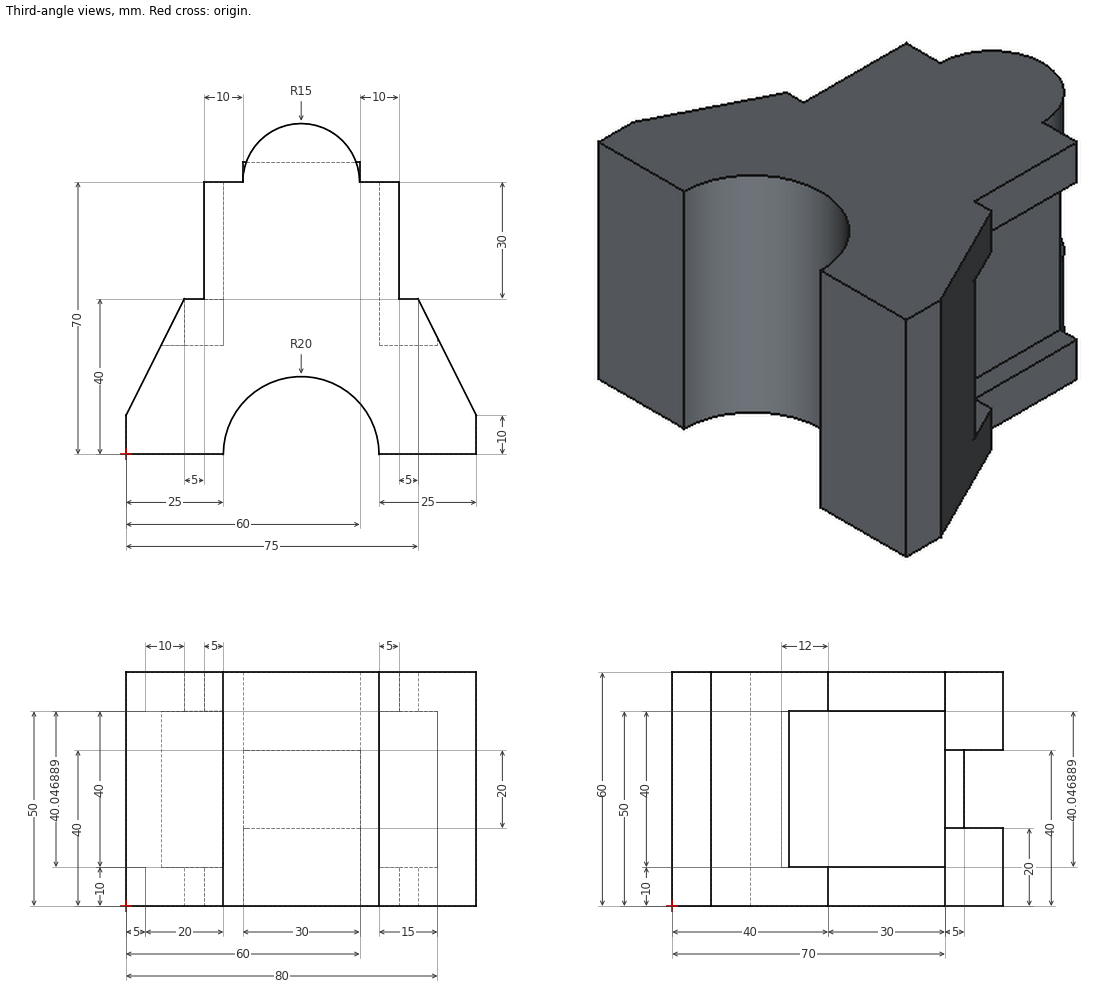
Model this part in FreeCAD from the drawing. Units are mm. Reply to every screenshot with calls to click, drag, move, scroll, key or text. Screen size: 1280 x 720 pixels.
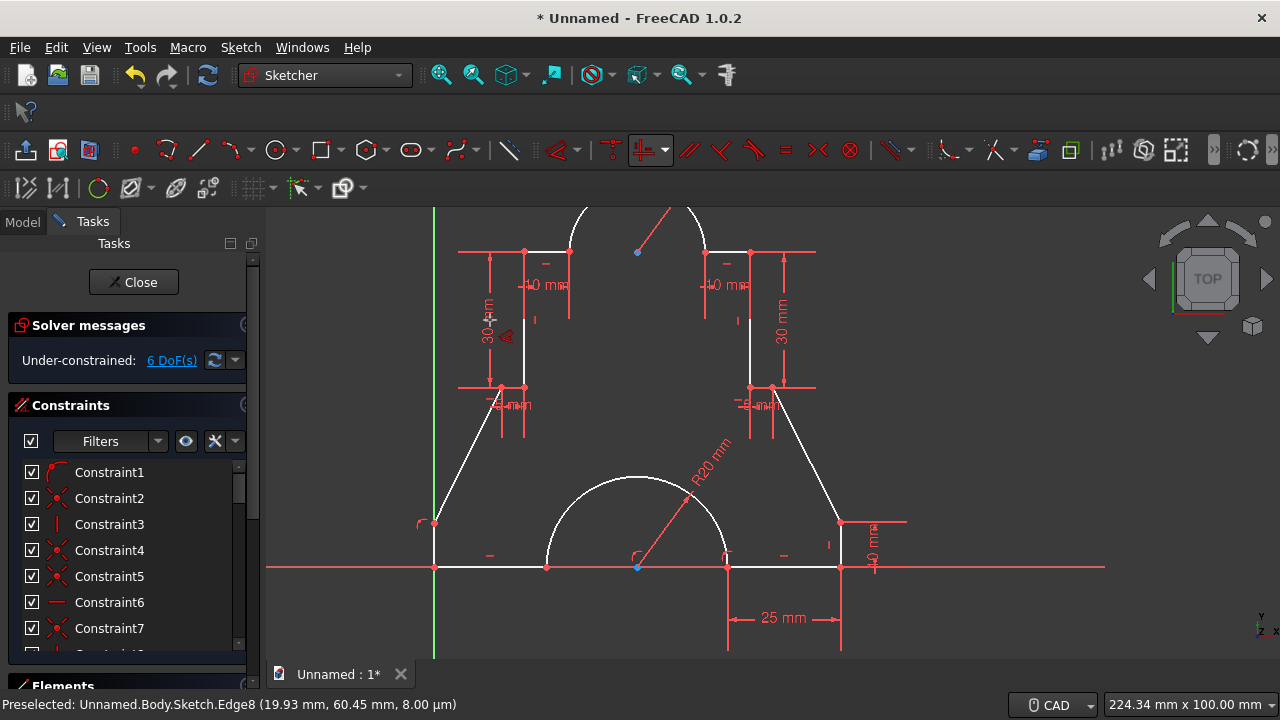
click(434, 536)
click(400, 545)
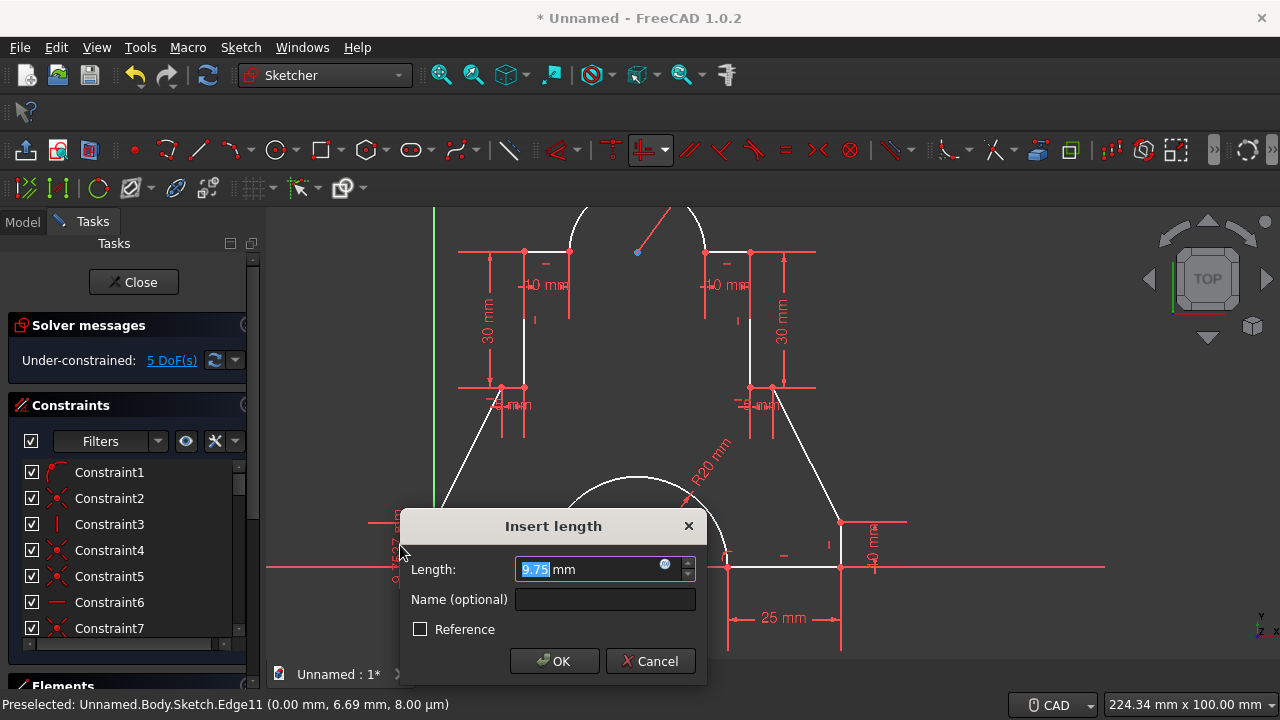
text(10)
key(Return)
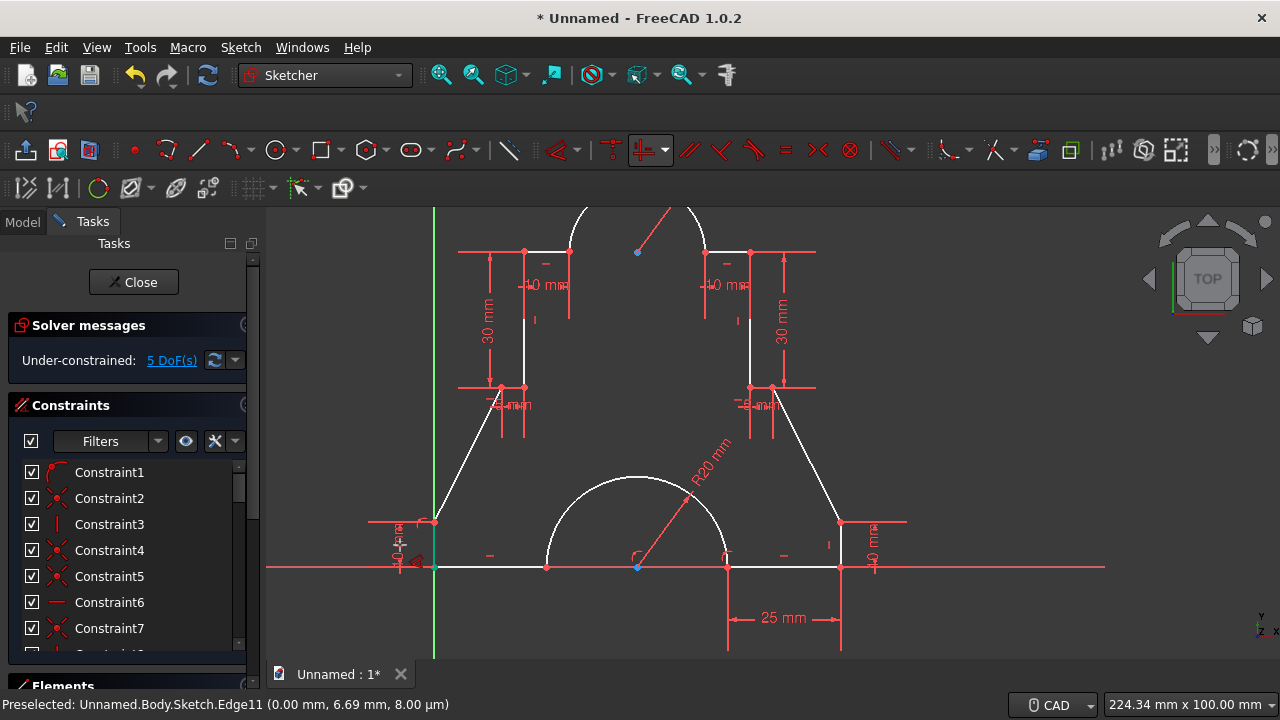
click(468, 567)
click(490, 601)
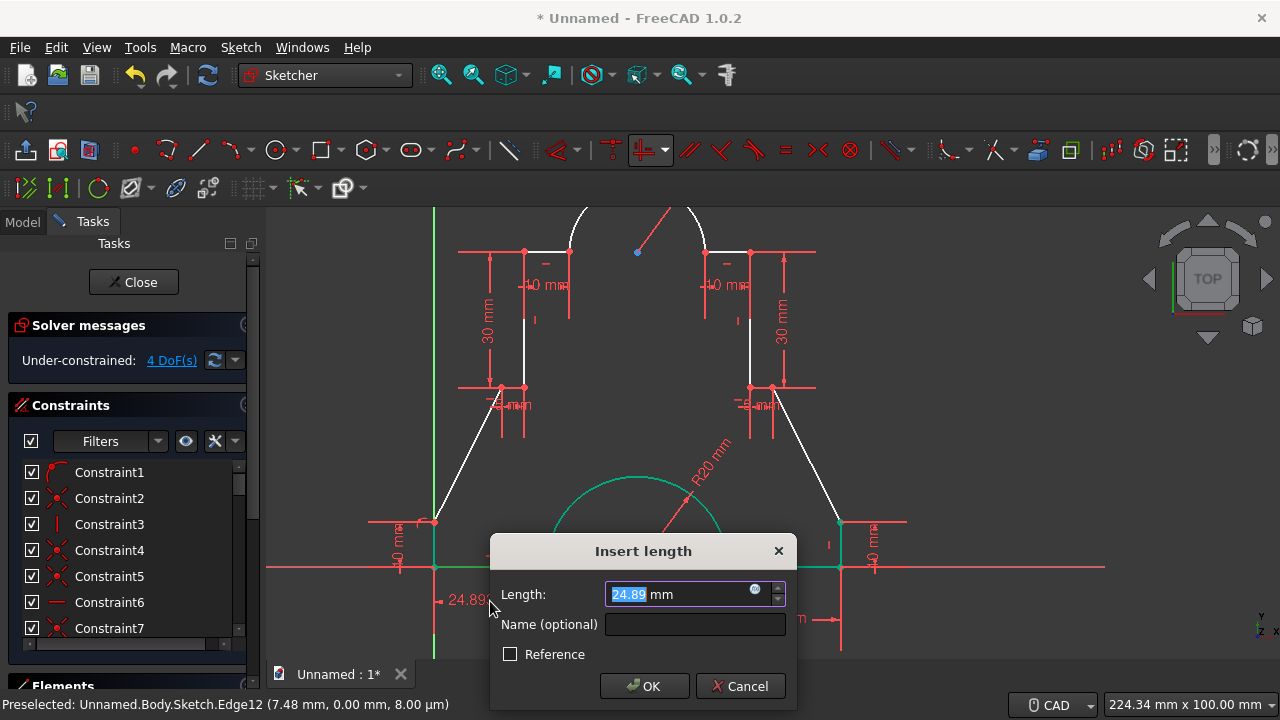
text(25)
key(Return)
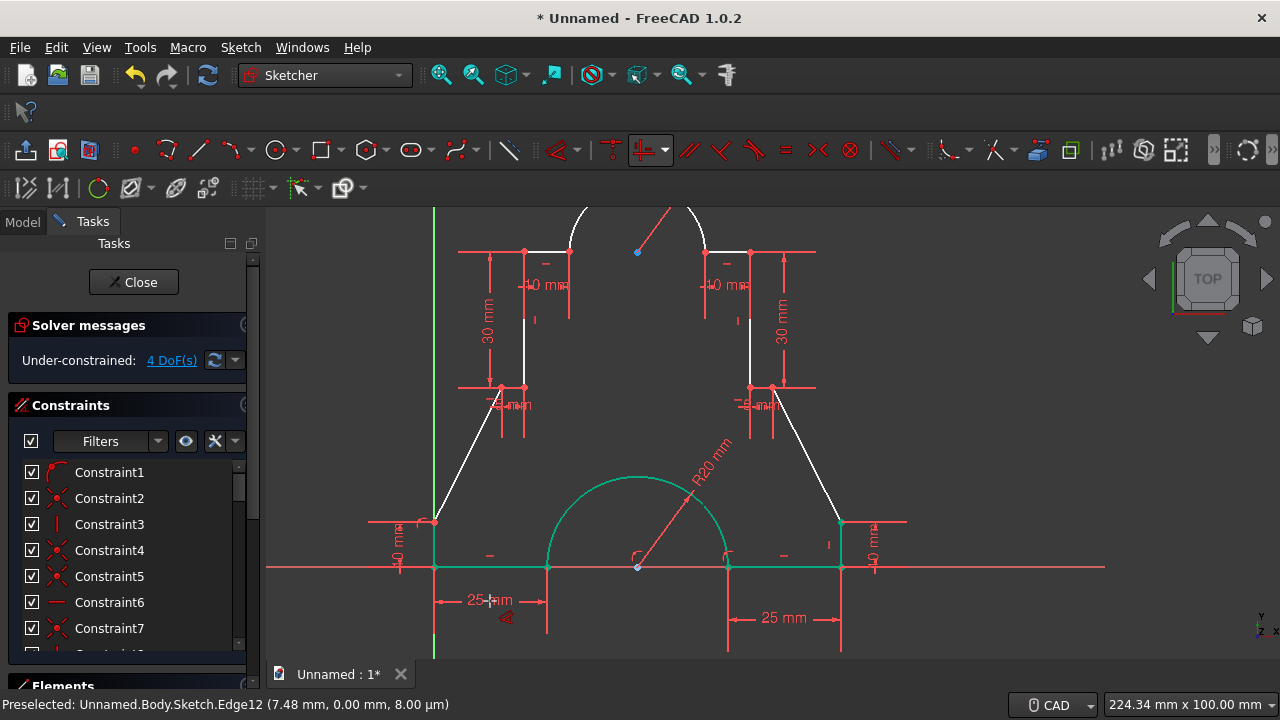
click(773, 388)
click(604, 601)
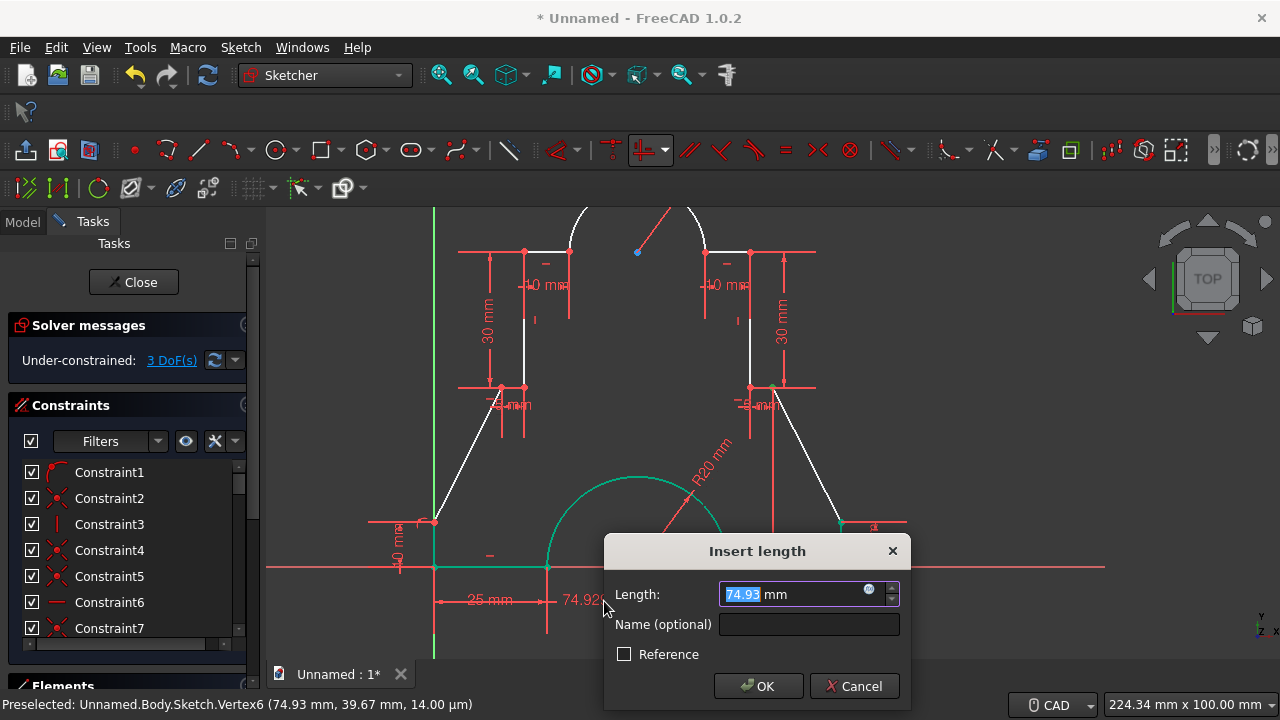
text(75)
key(Return)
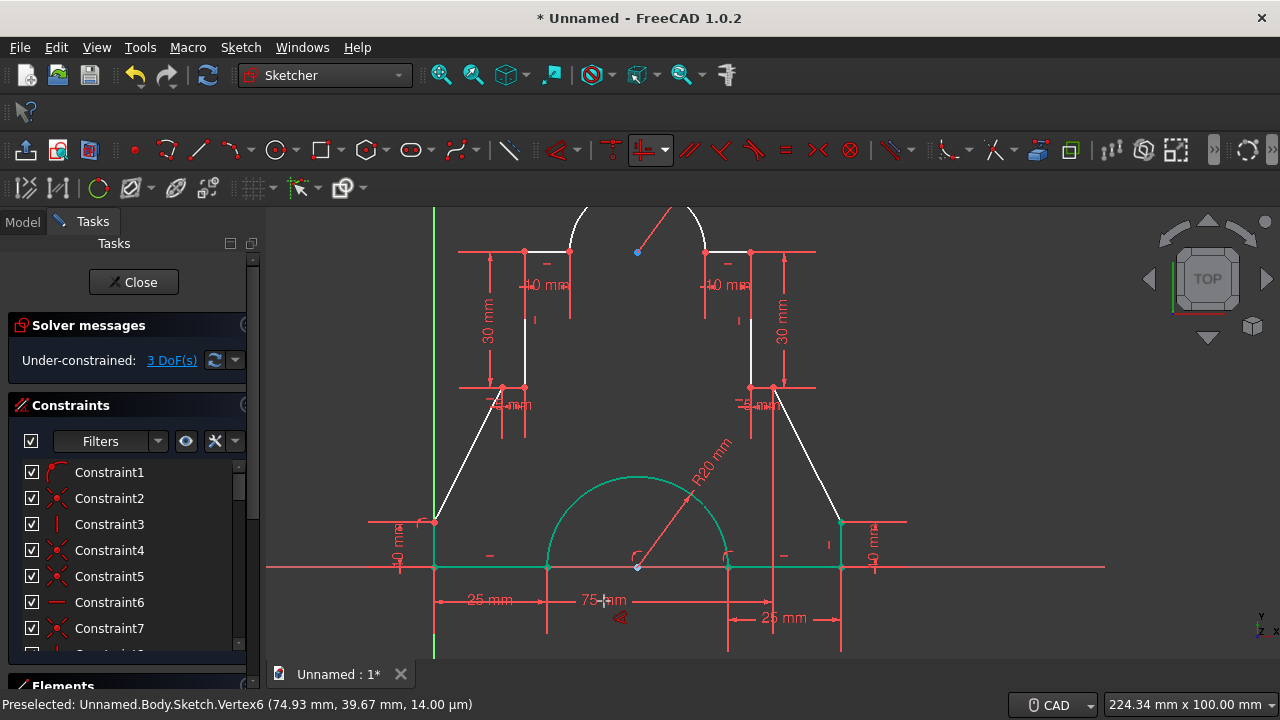
click(773, 388)
click(400, 478)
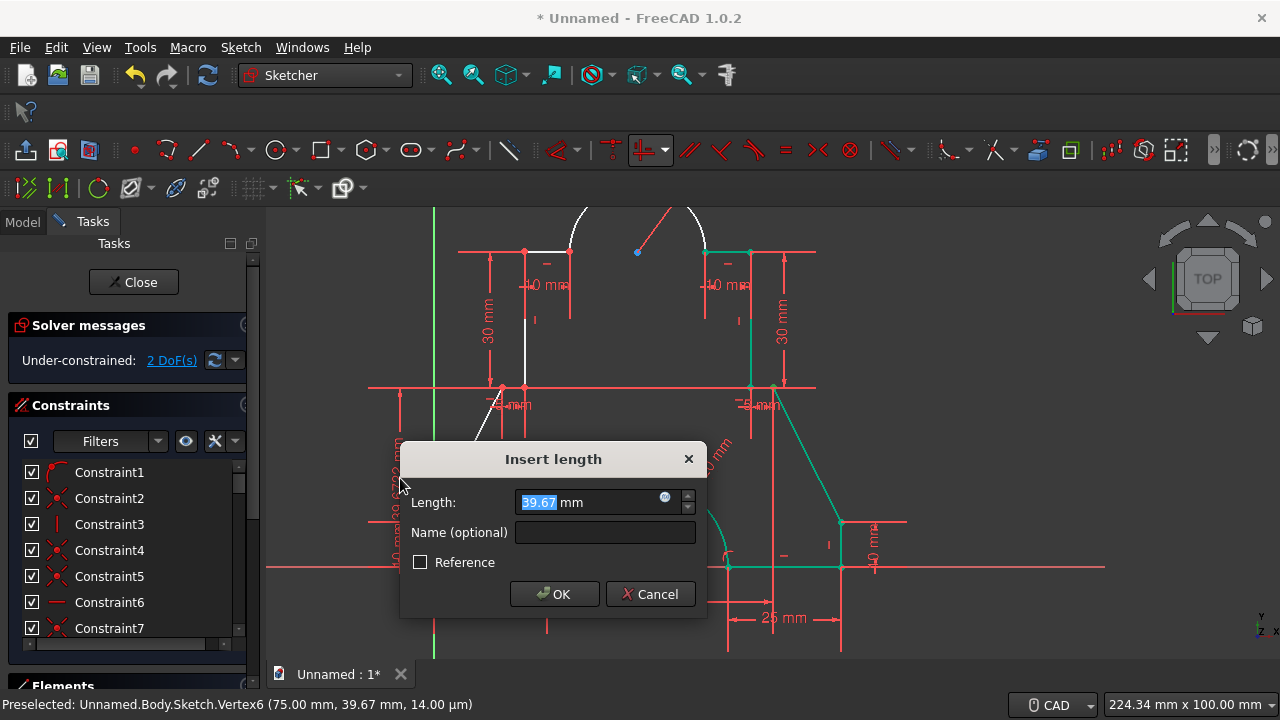
text(40)
key(Return)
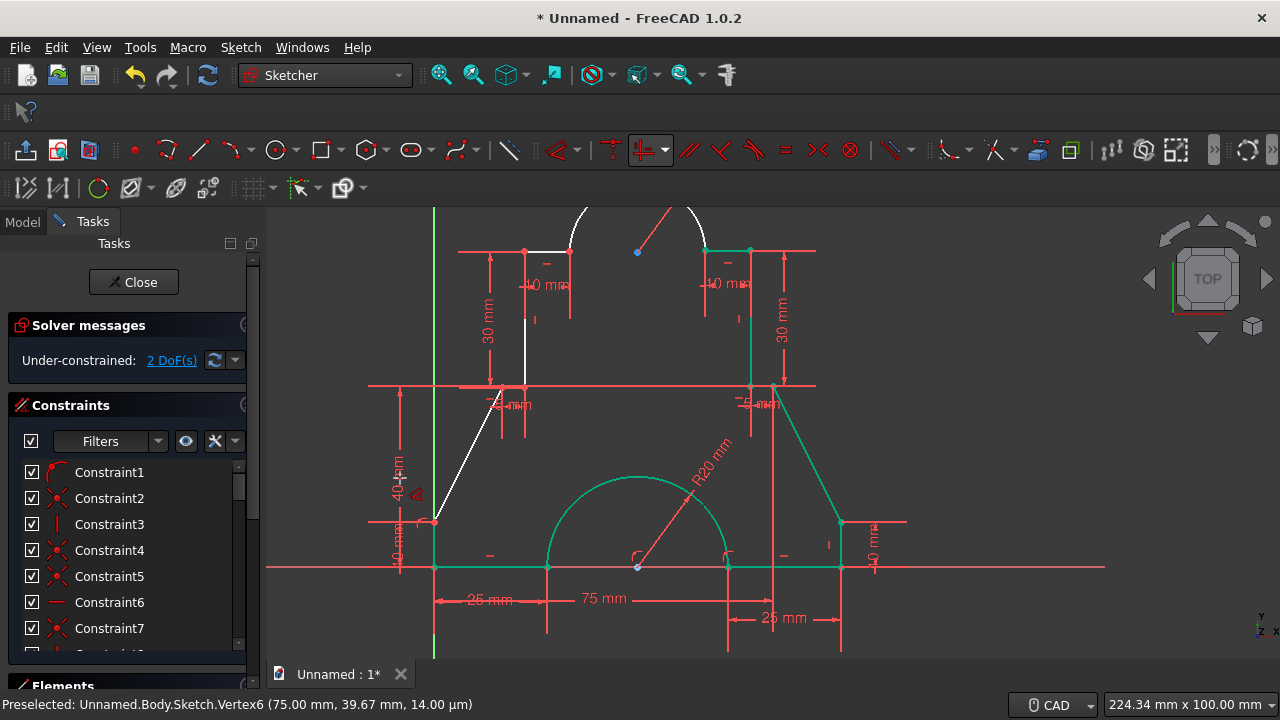
click(570, 252)
click(400, 410)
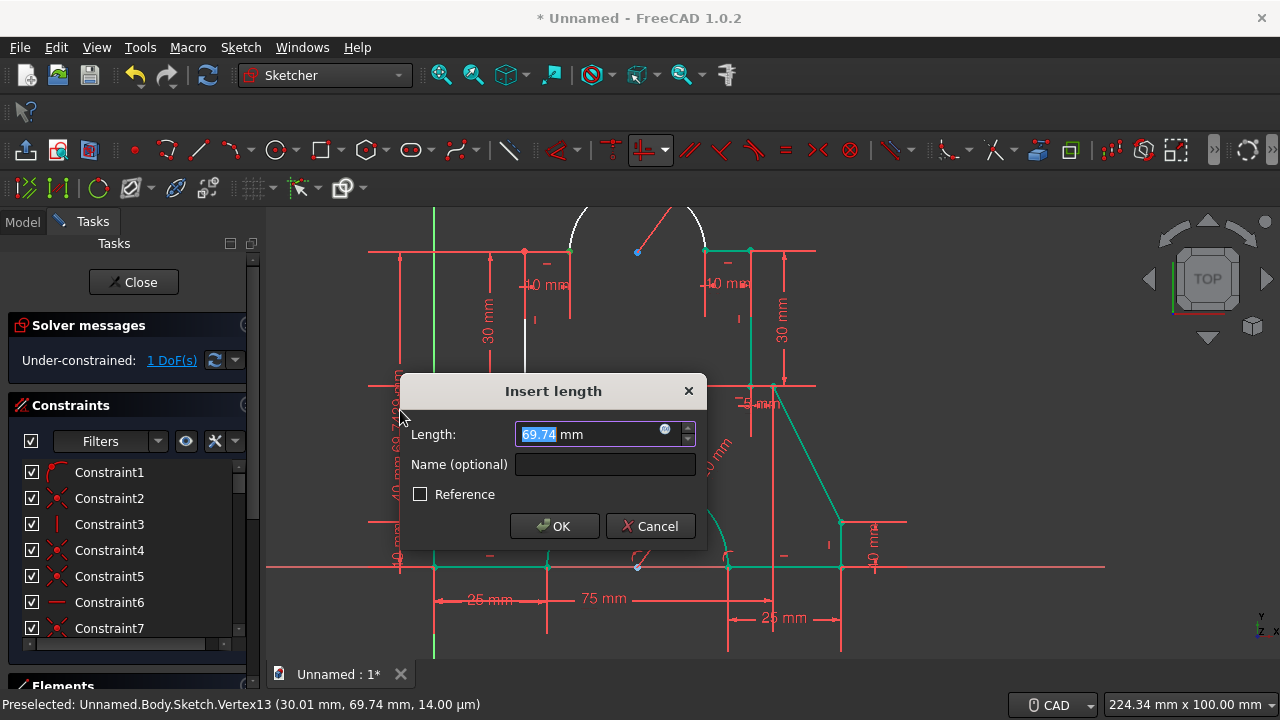
text(70)
key(Return)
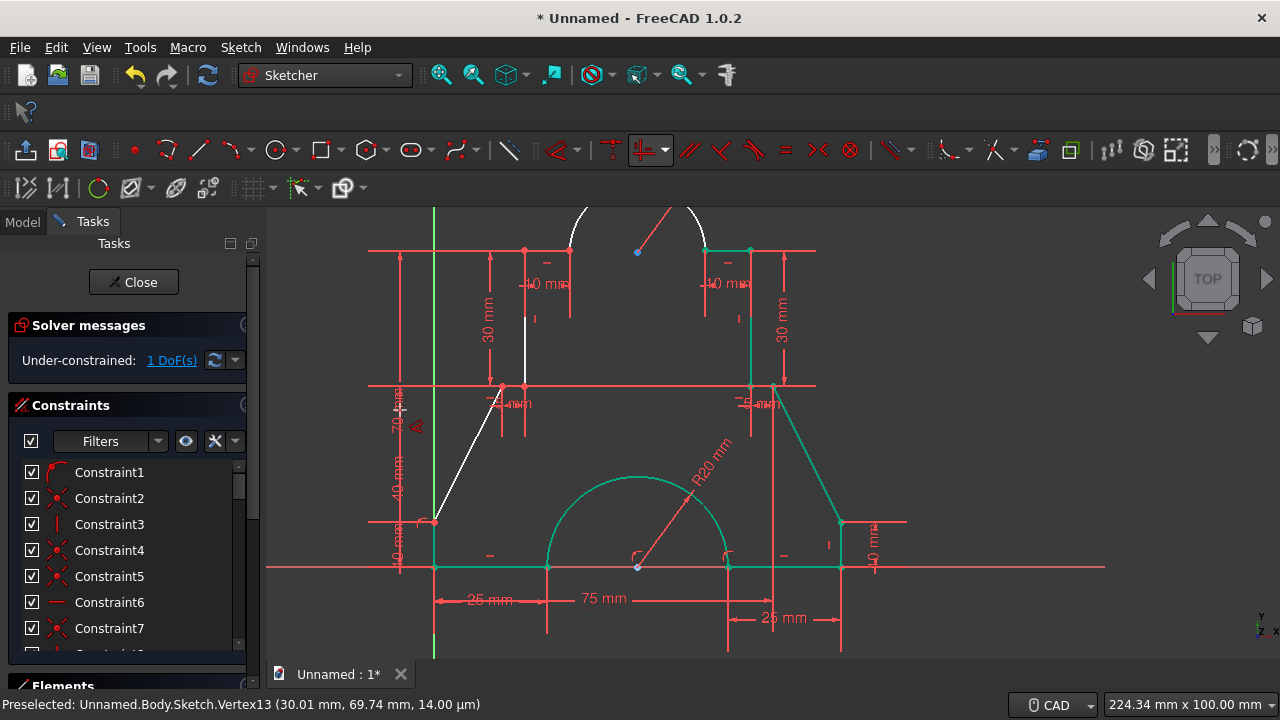
click(638, 253)
click(400, 338)